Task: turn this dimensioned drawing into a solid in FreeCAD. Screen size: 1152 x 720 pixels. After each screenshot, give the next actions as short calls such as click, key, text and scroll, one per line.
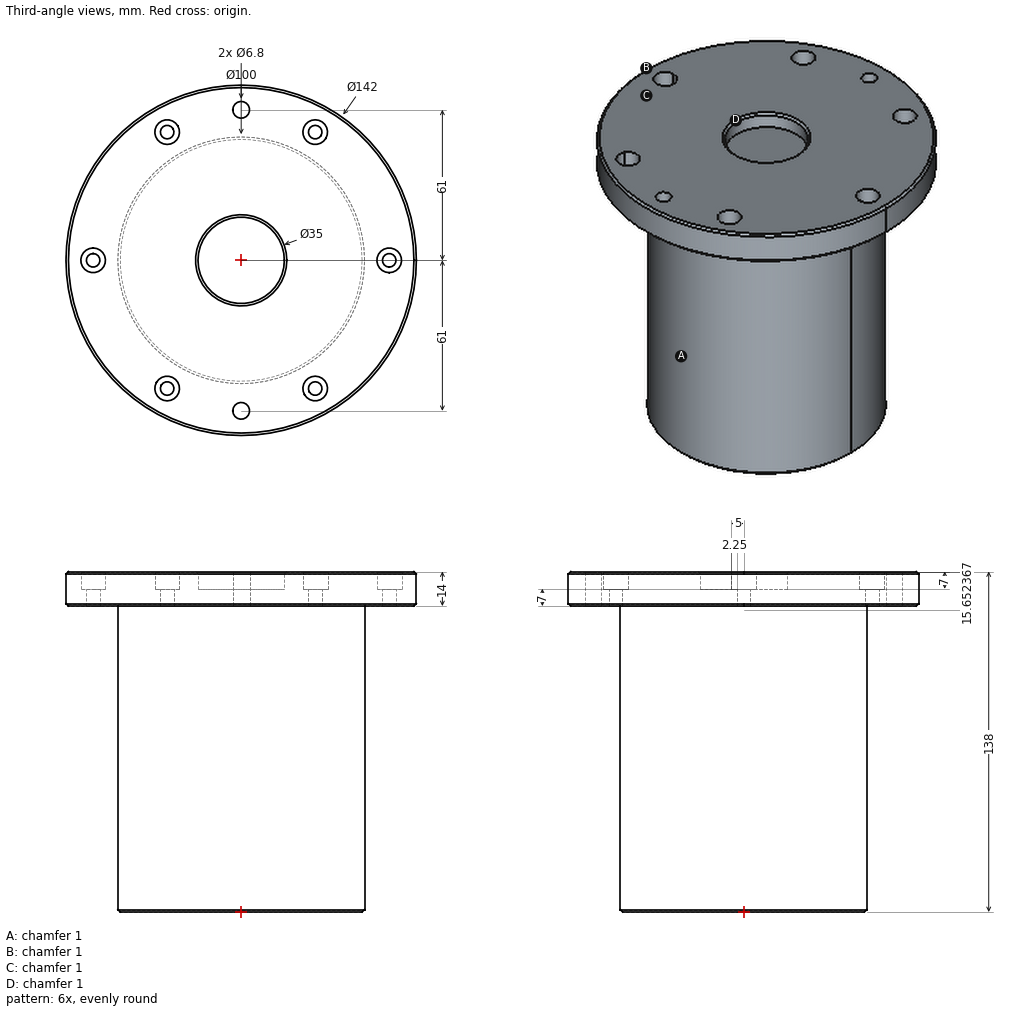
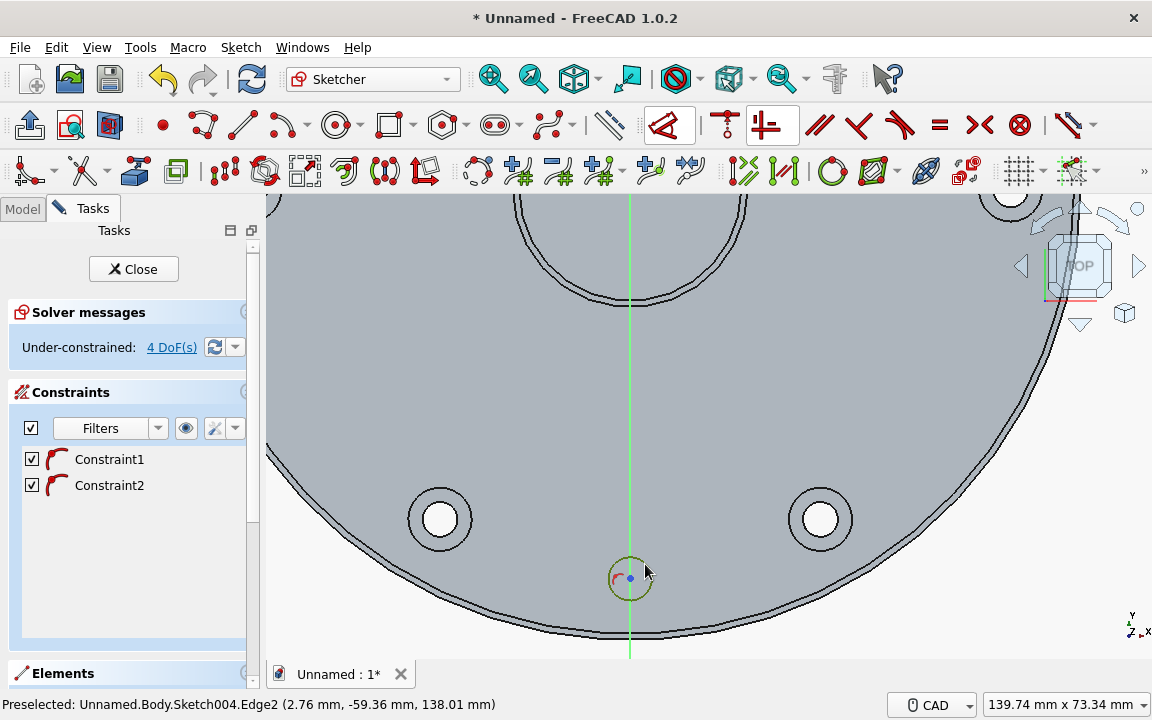
key(e)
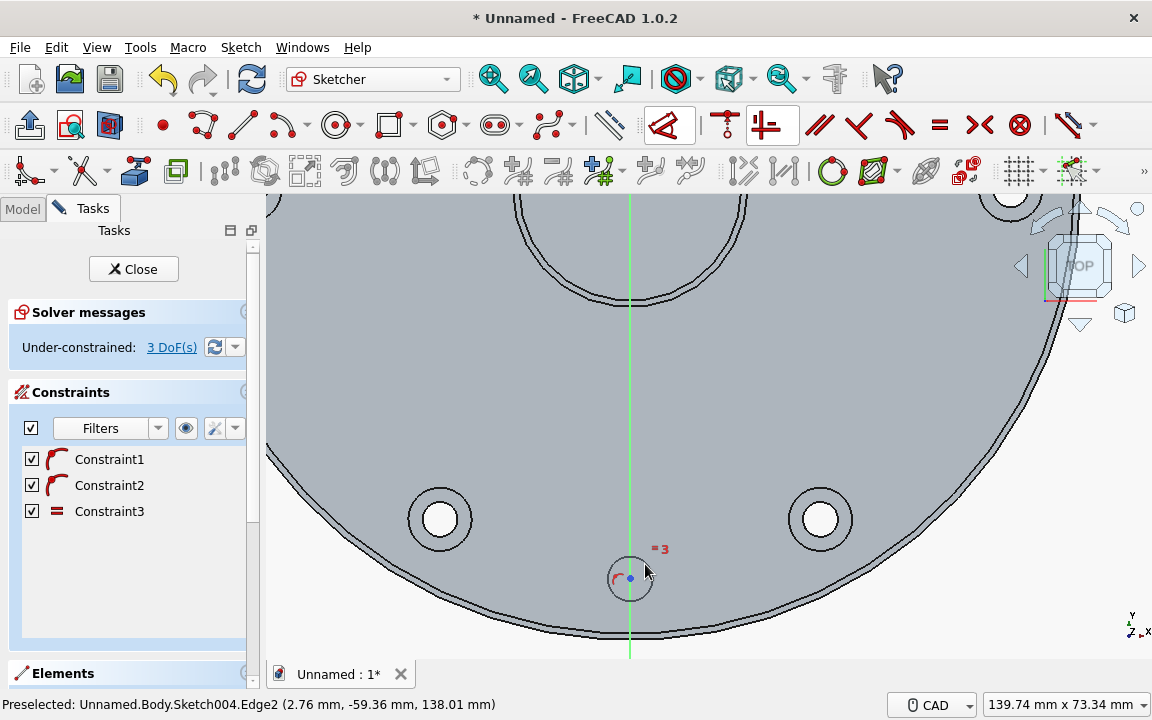
scroll(646, 564, down, 5)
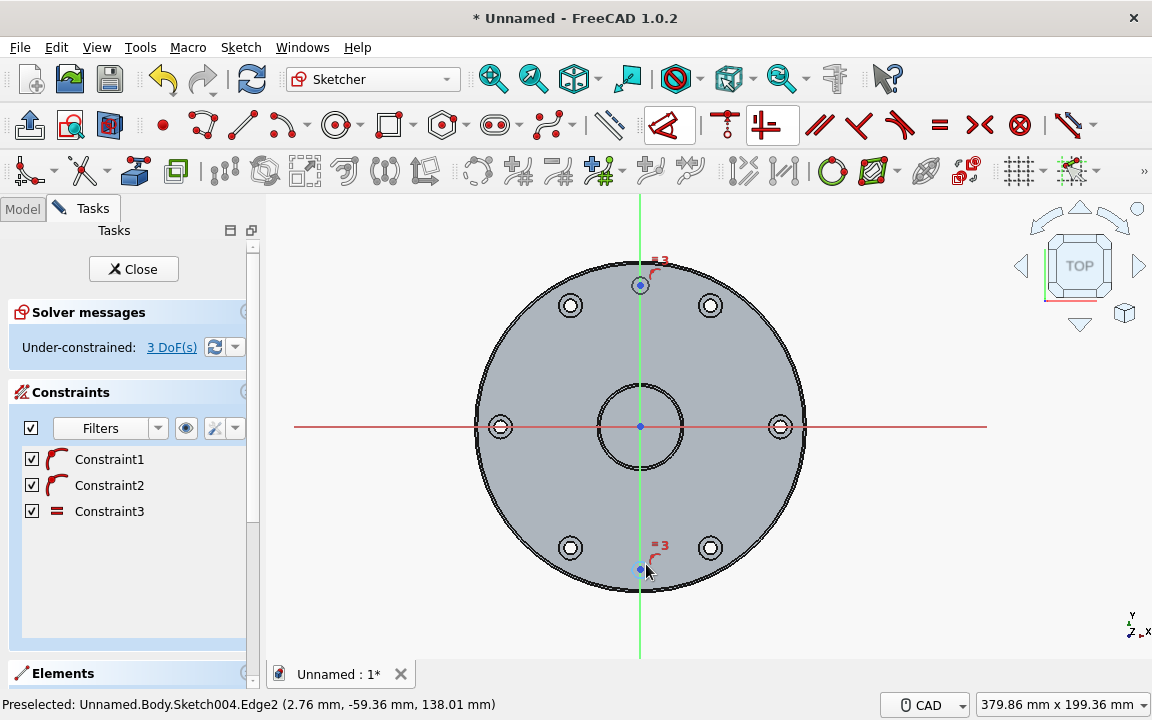
scroll(646, 280, up, 5)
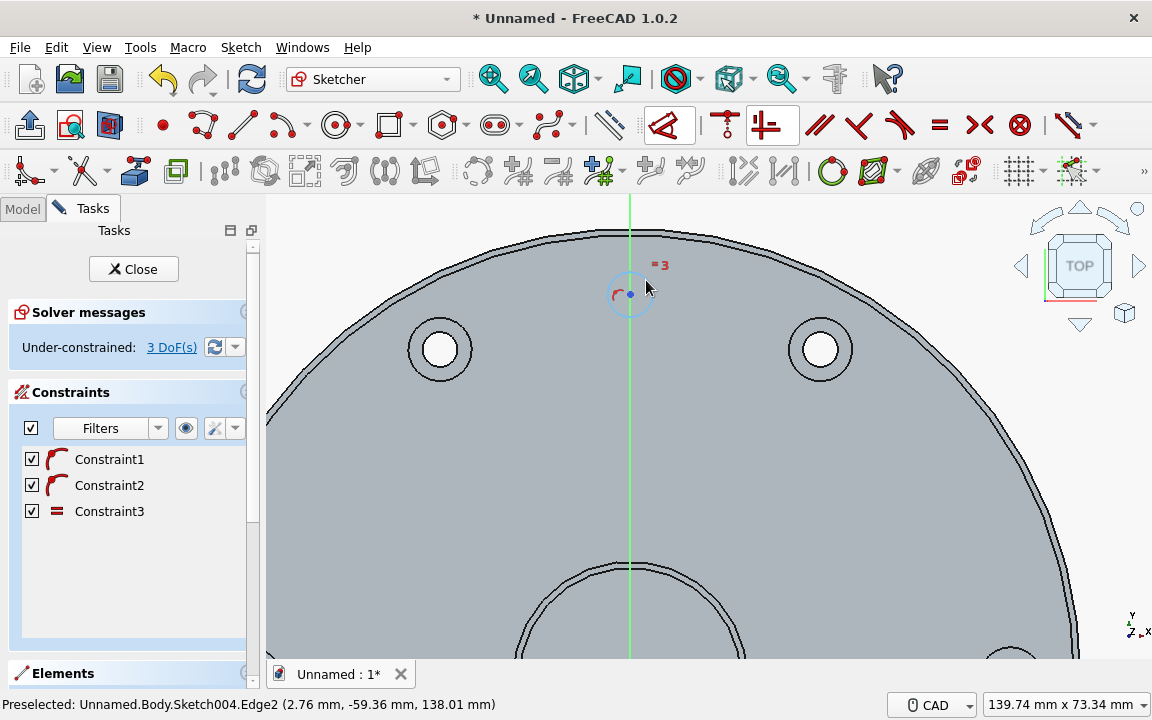
click(646, 279)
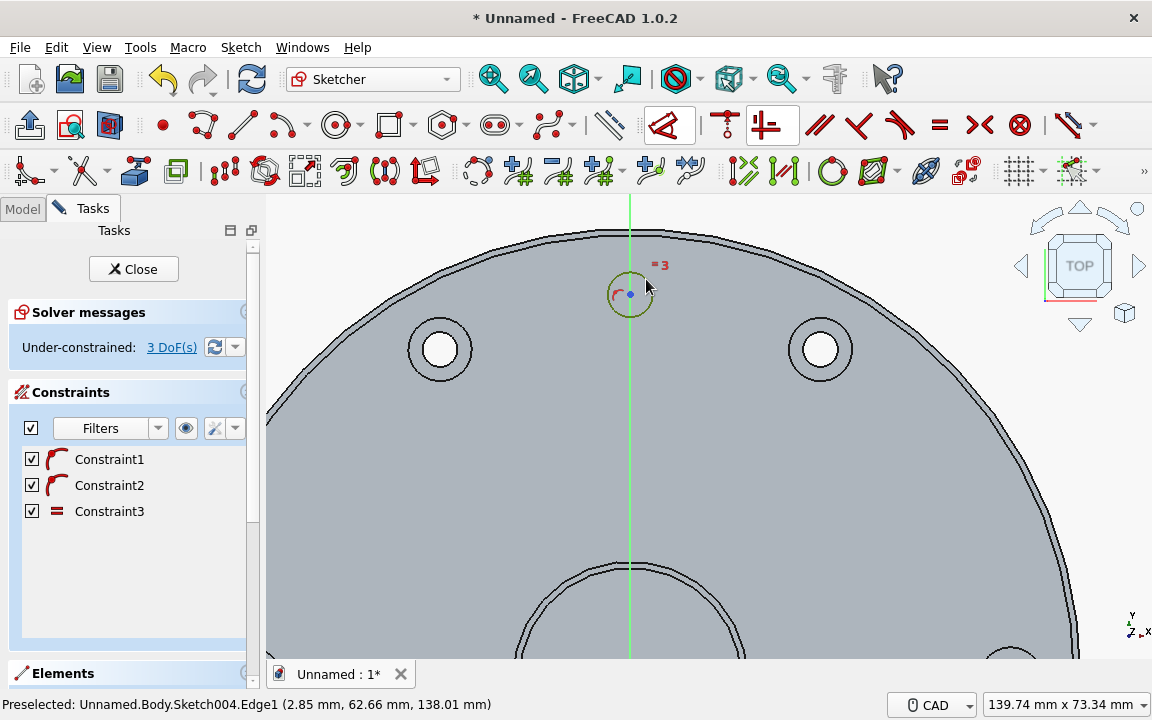
key(k)
key(o)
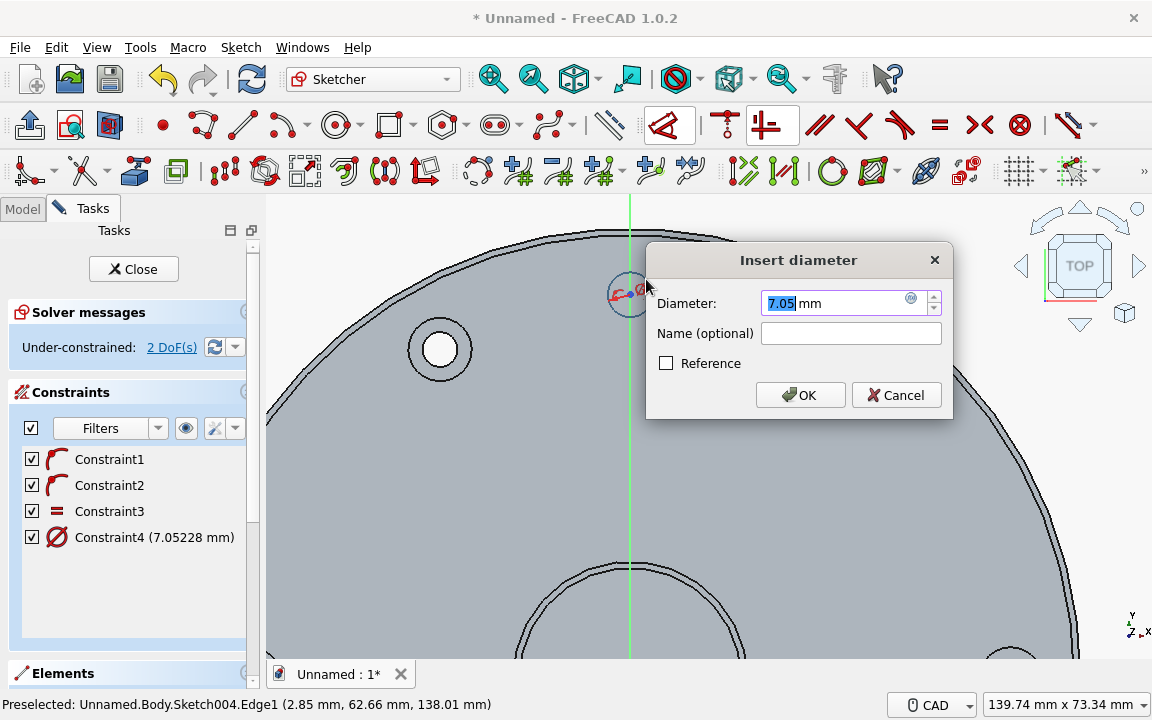
text(6.8)
key(Return)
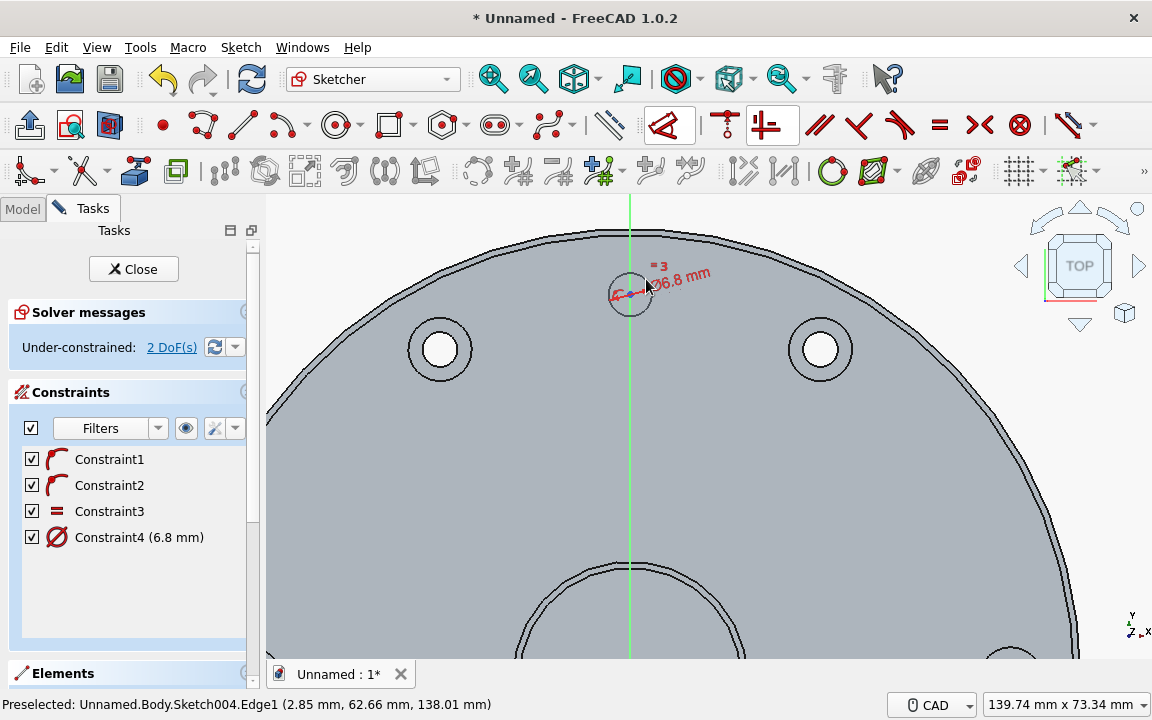
click(630, 295)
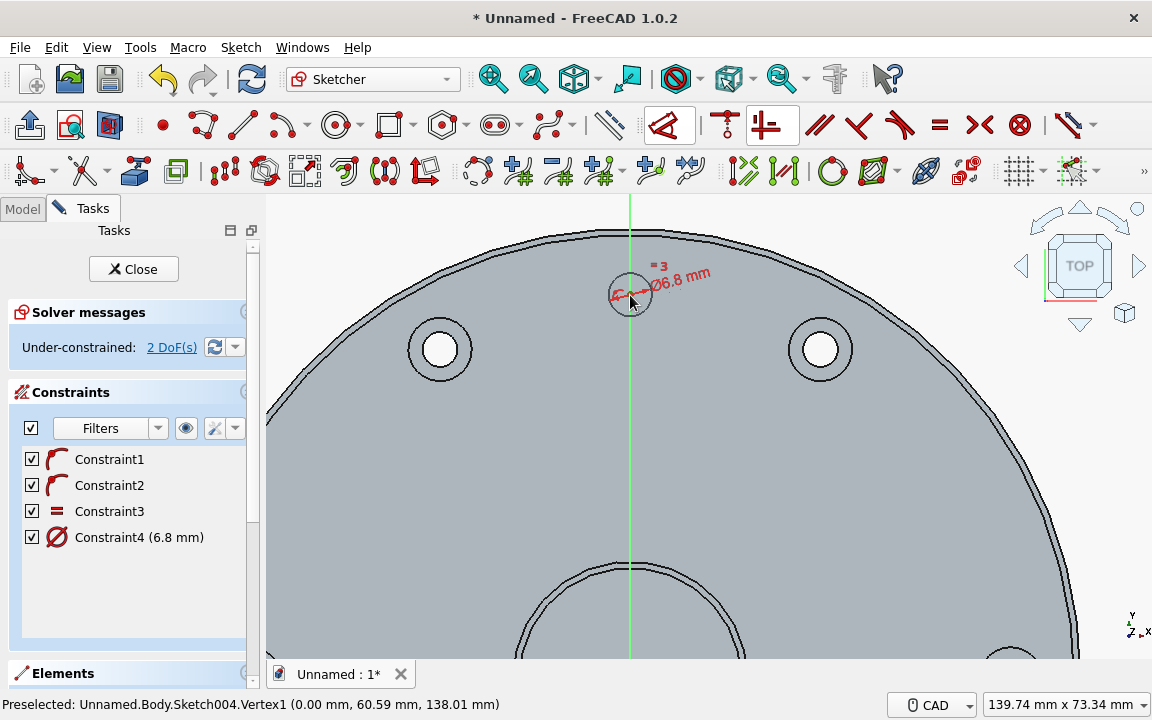
key(i)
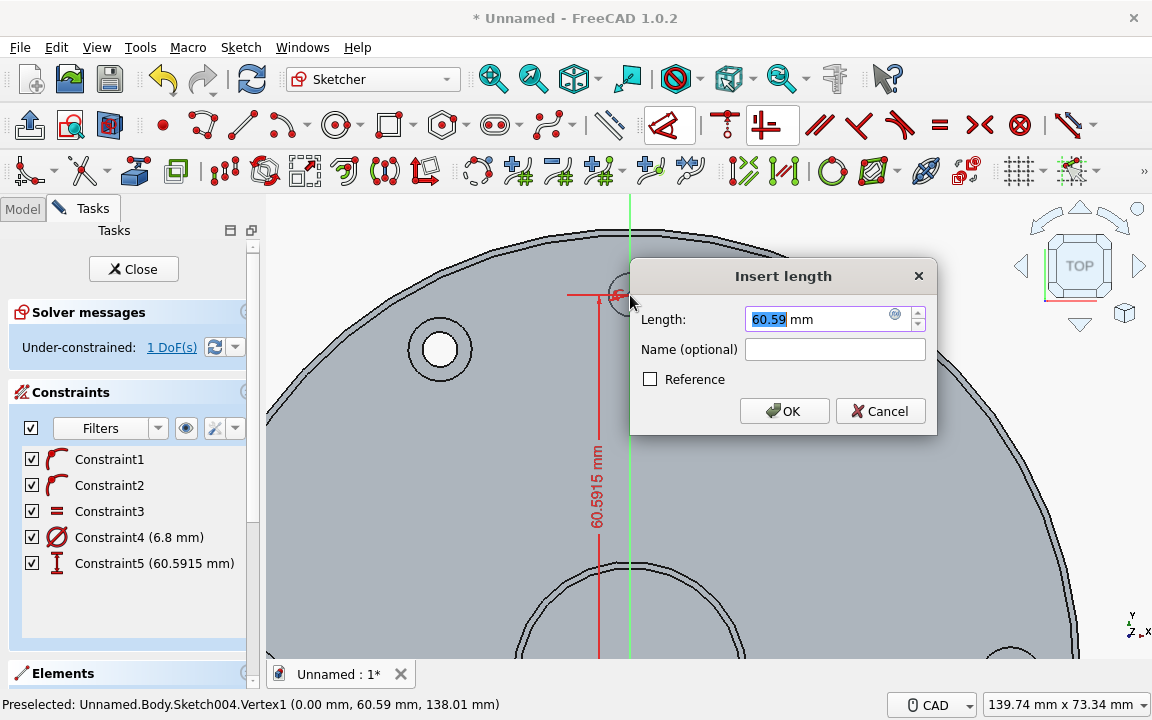
text(61)
key(Return)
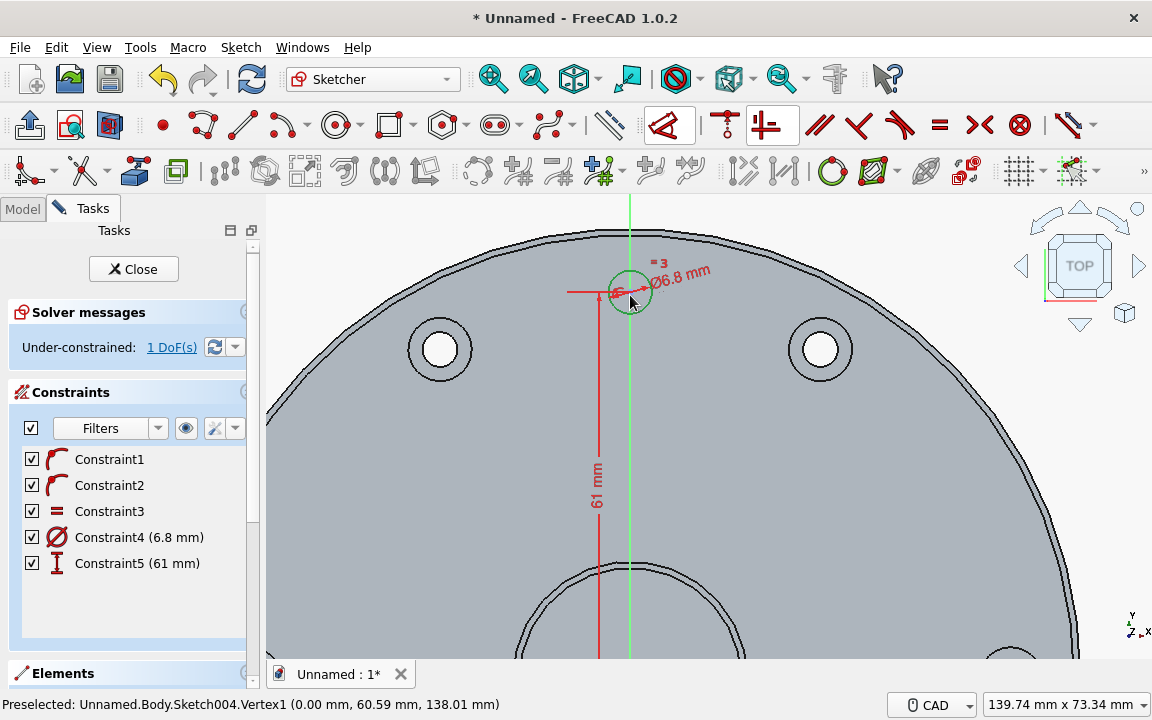
scroll(646, 280, down, 5)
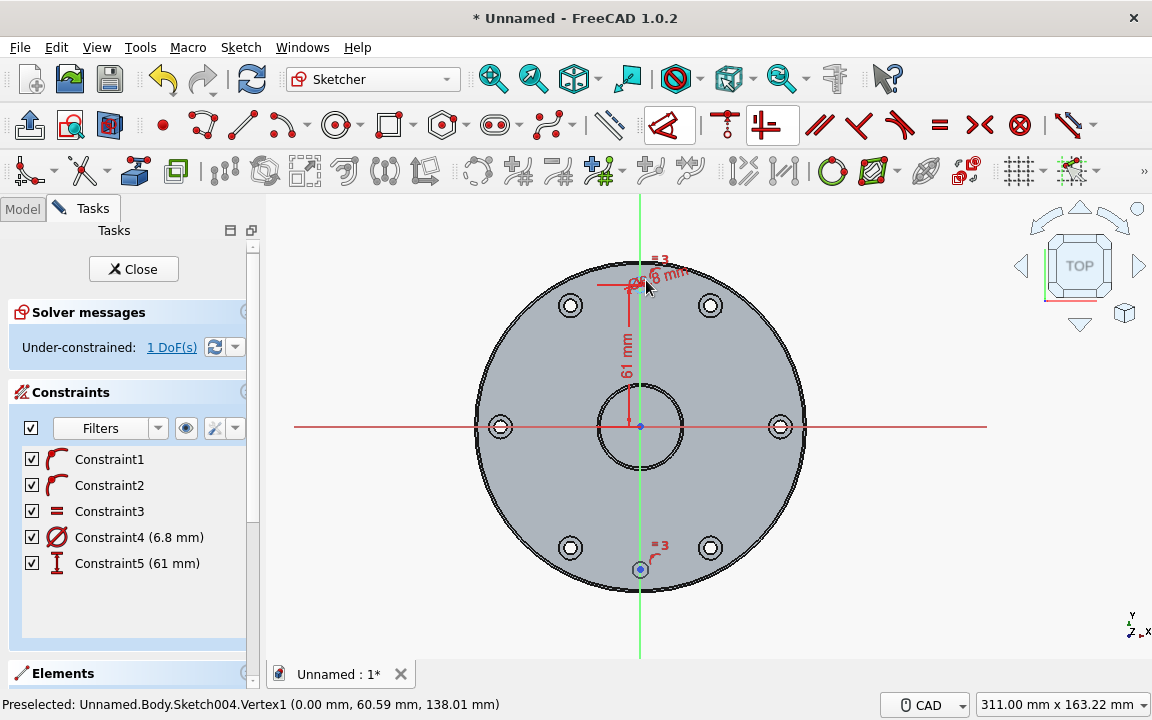
click(640, 570)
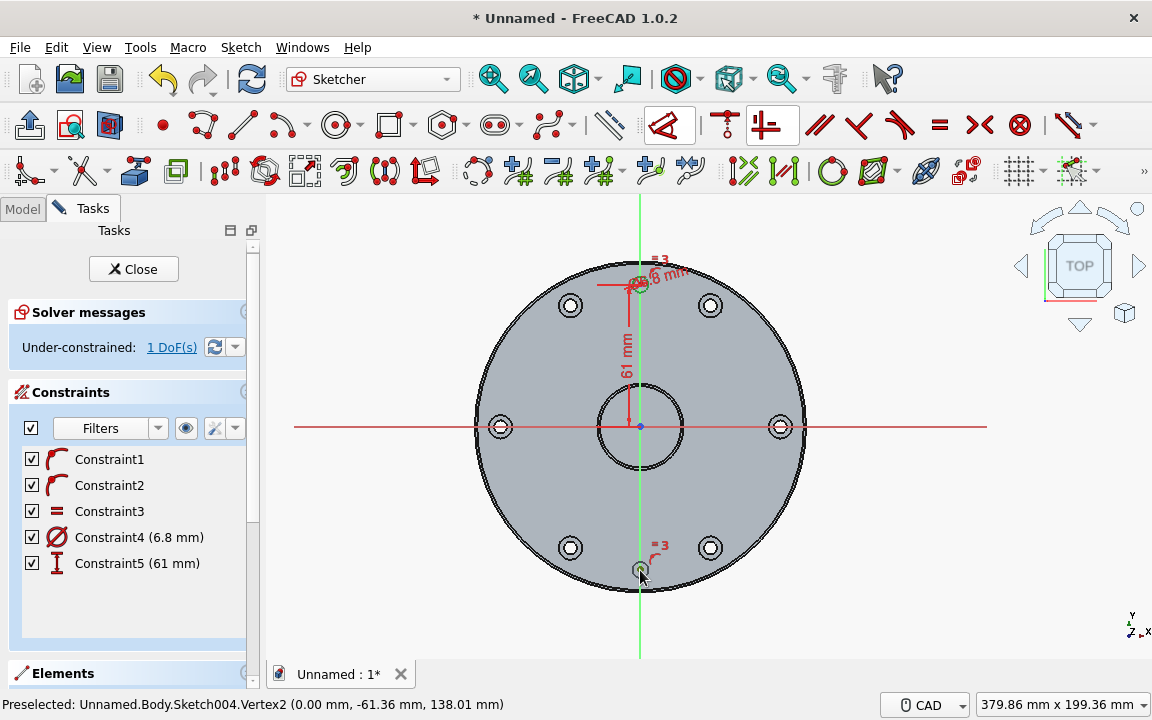
key(i)